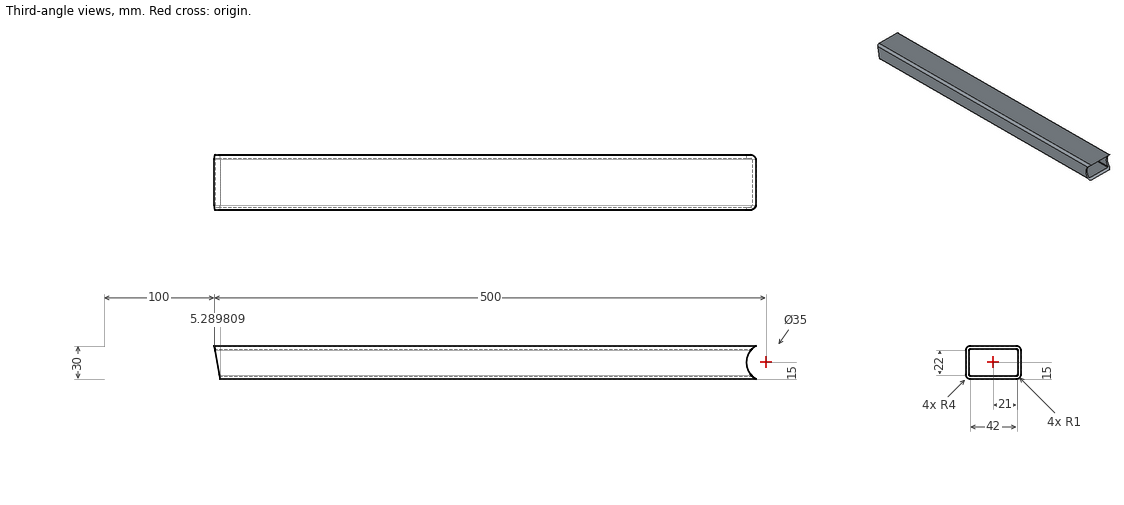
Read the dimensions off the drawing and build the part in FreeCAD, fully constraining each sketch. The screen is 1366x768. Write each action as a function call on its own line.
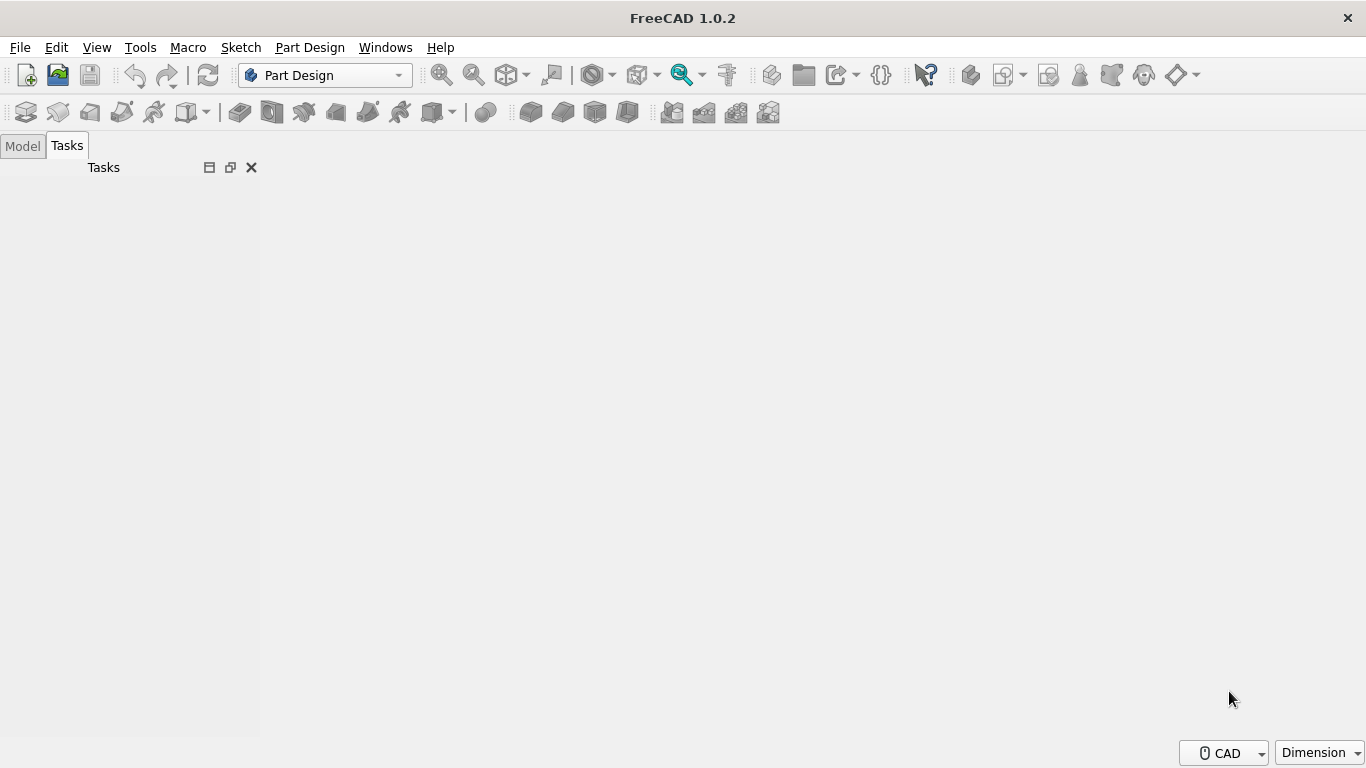
key(ctrl+n)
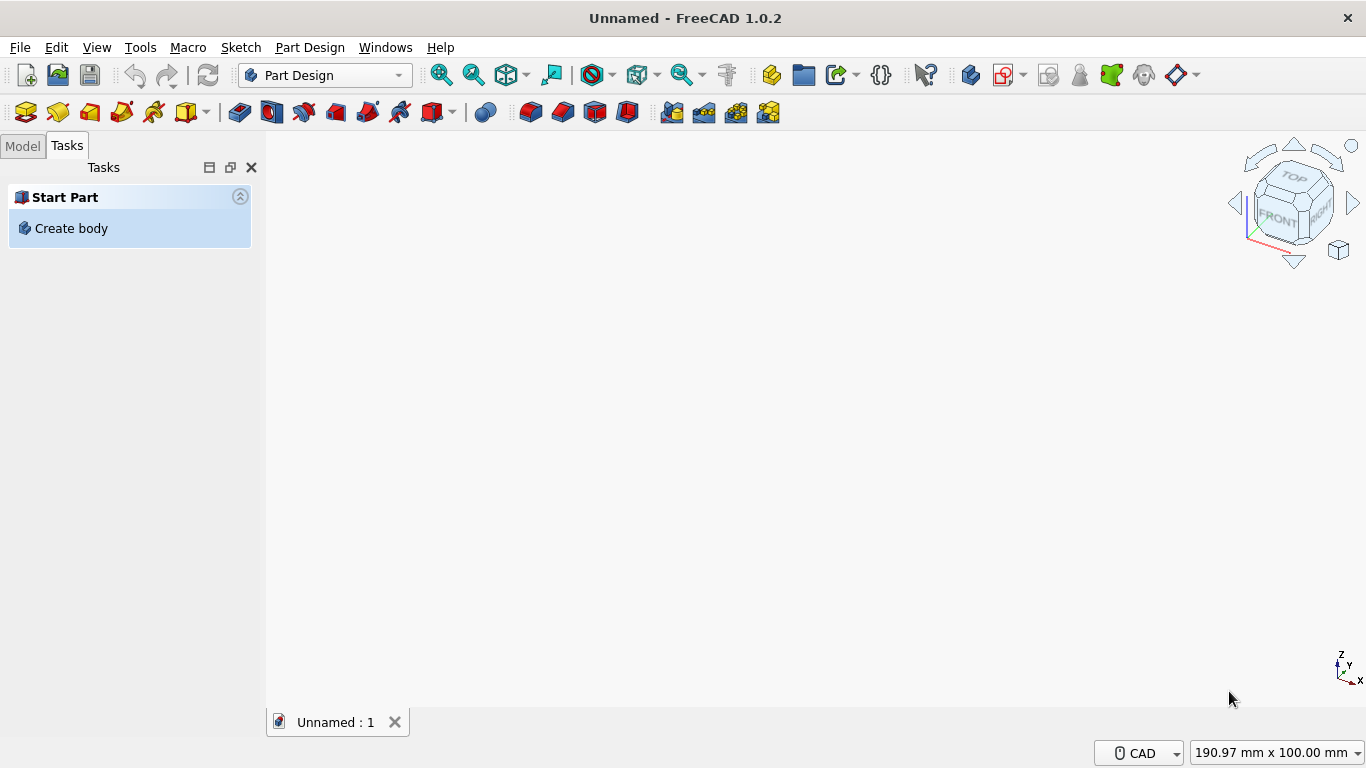
click(1004, 76)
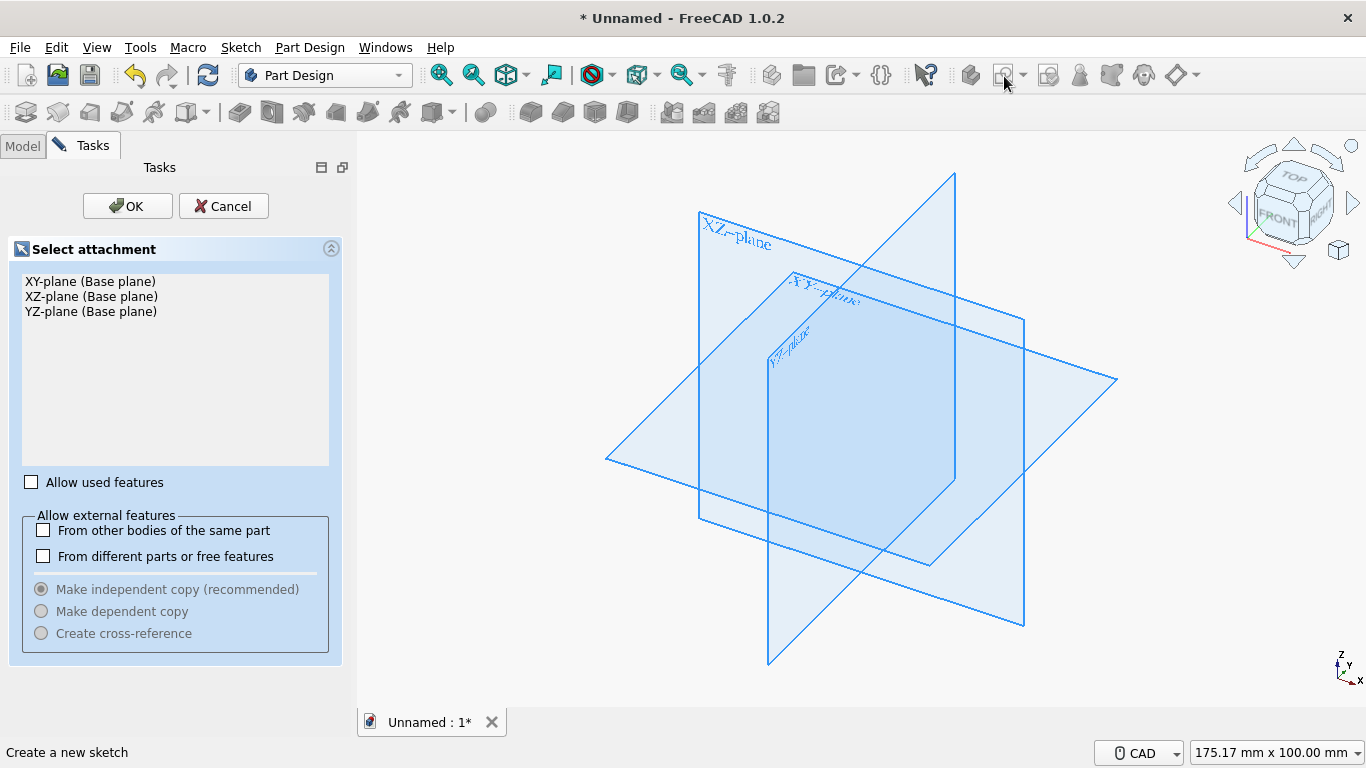
click(82, 312)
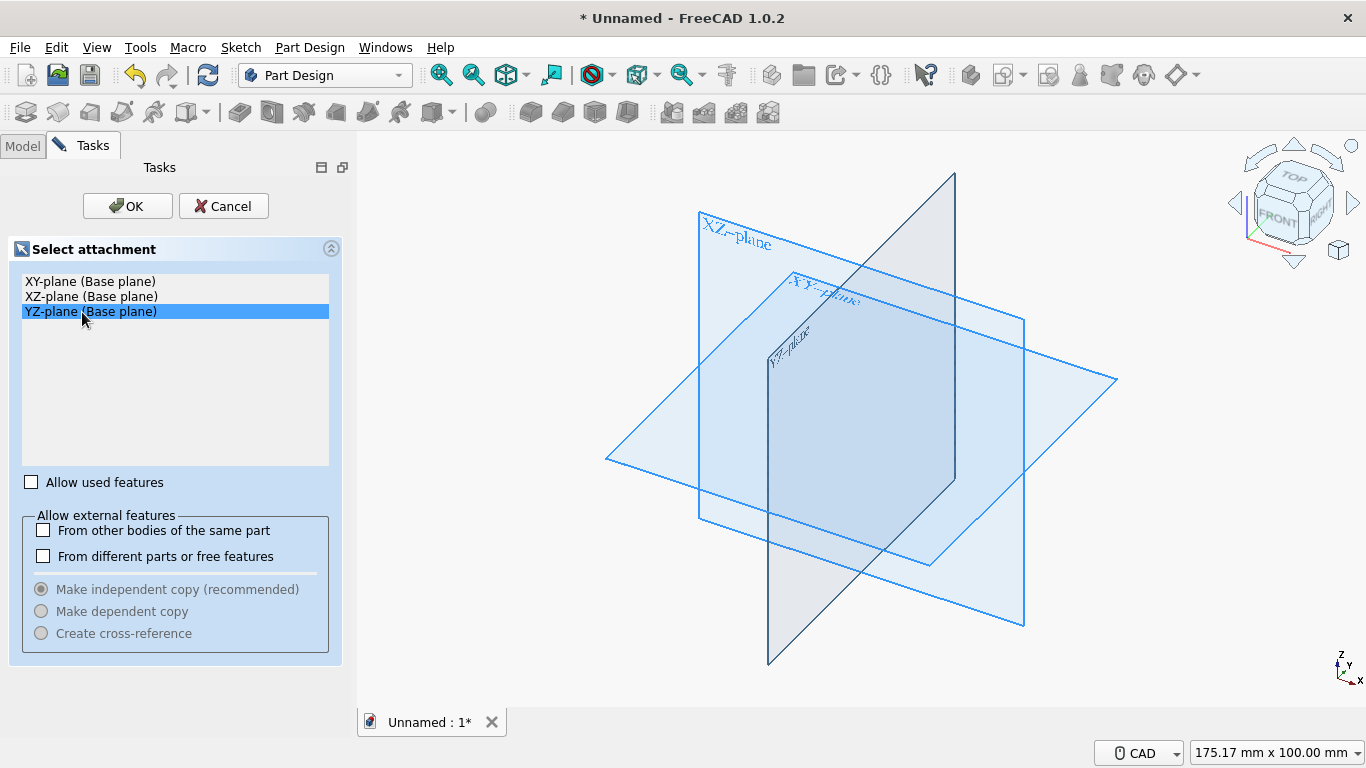
click(128, 206)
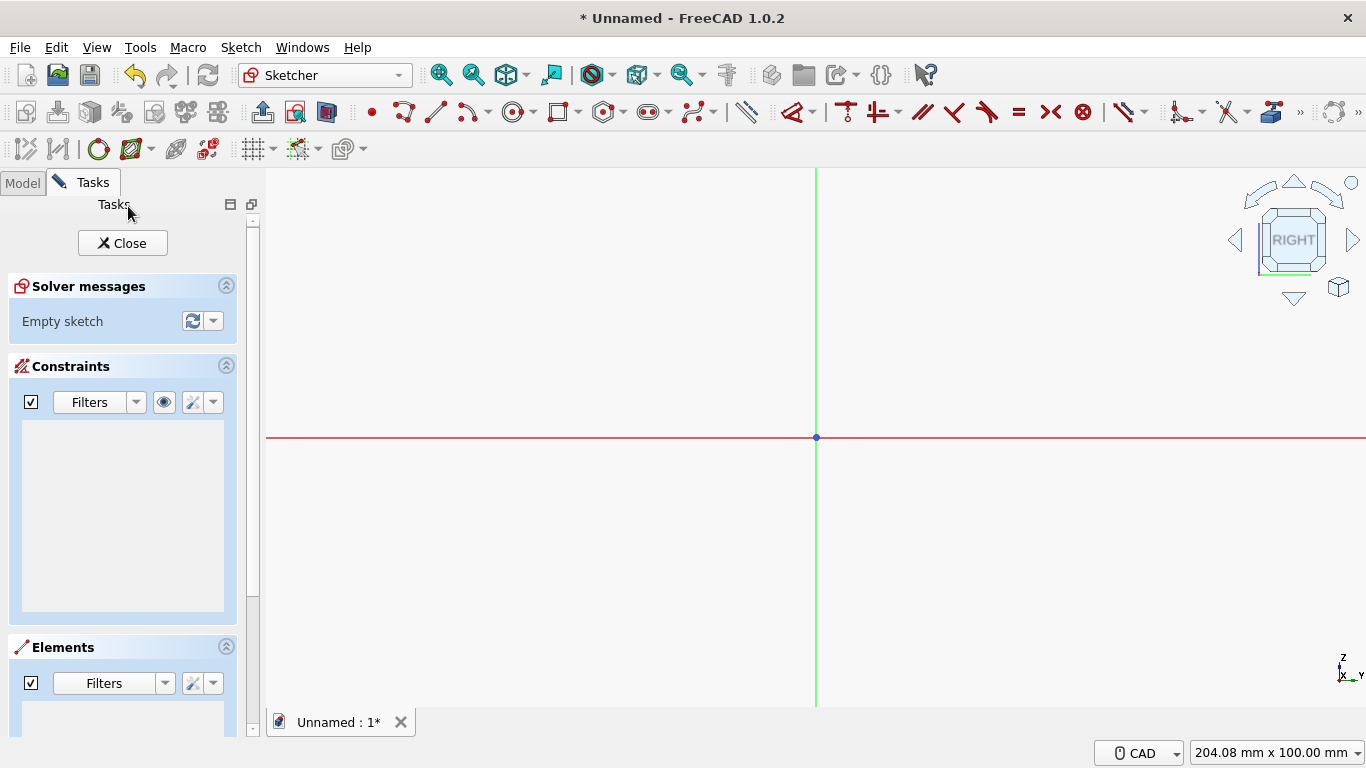
scroll(872, 438, up, 4)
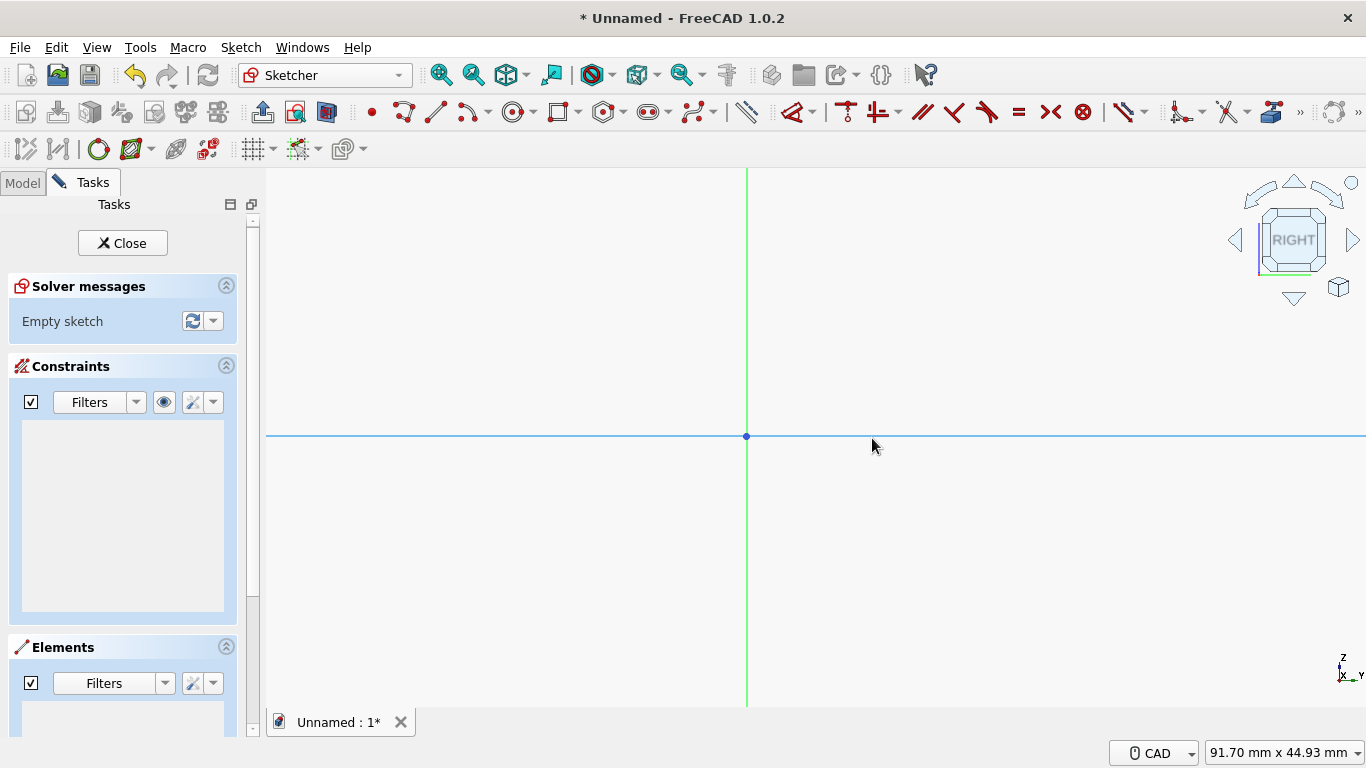
key(g)
key(l)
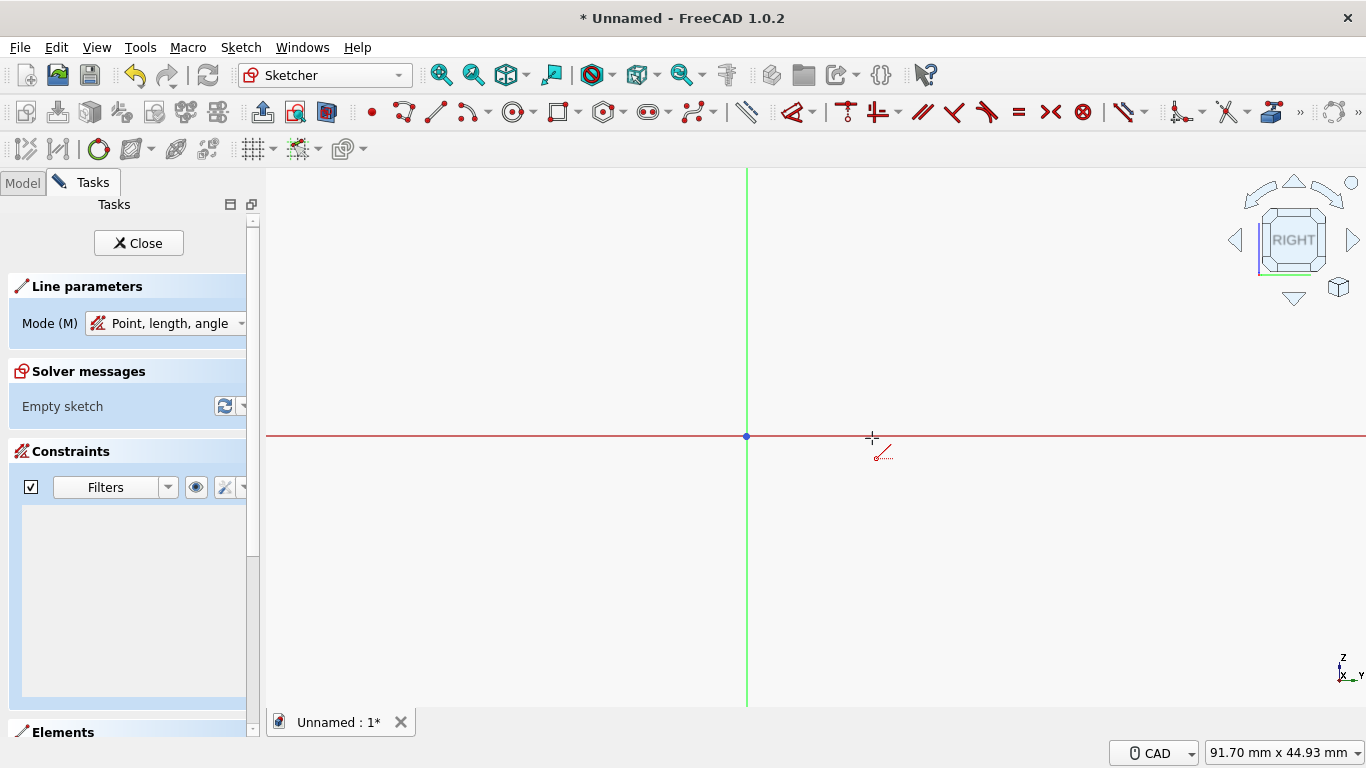
click(999, 616)
click(495, 616)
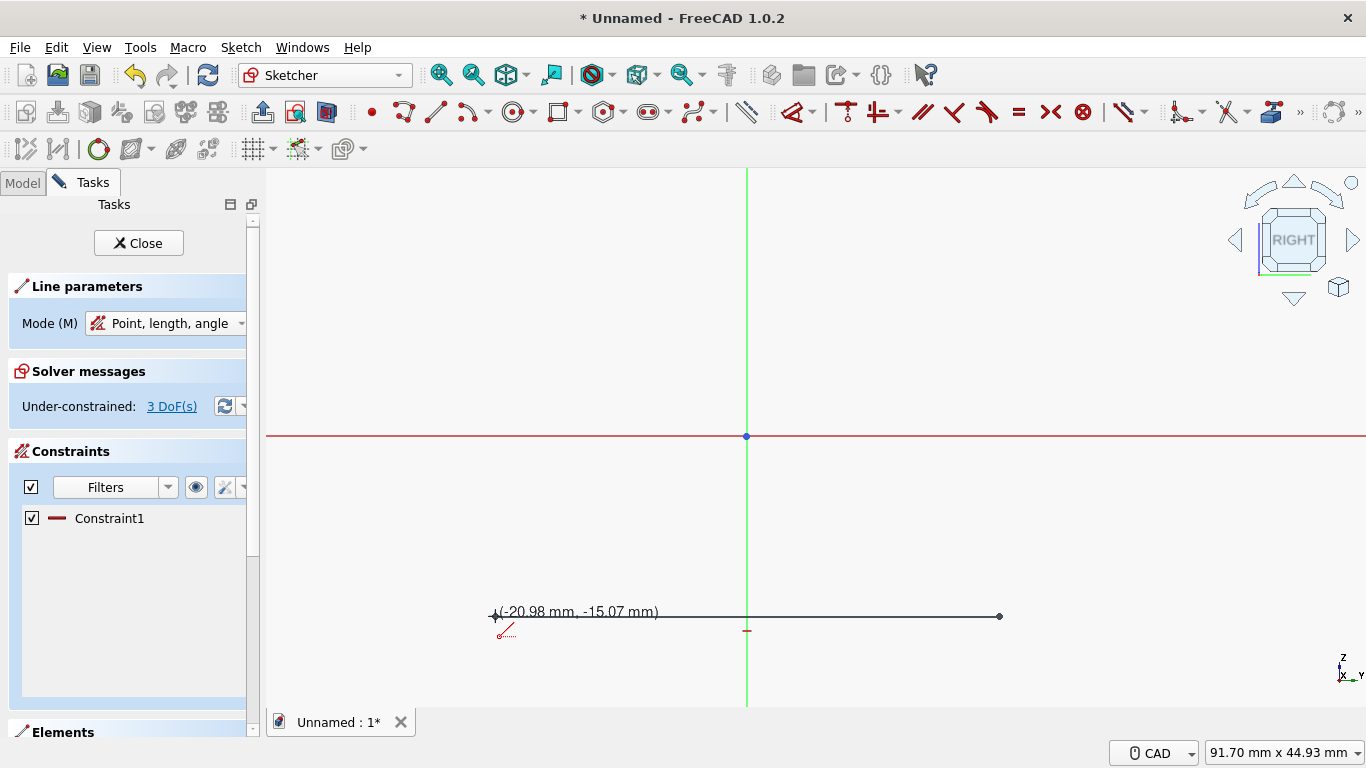
click(447, 568)
click(447, 304)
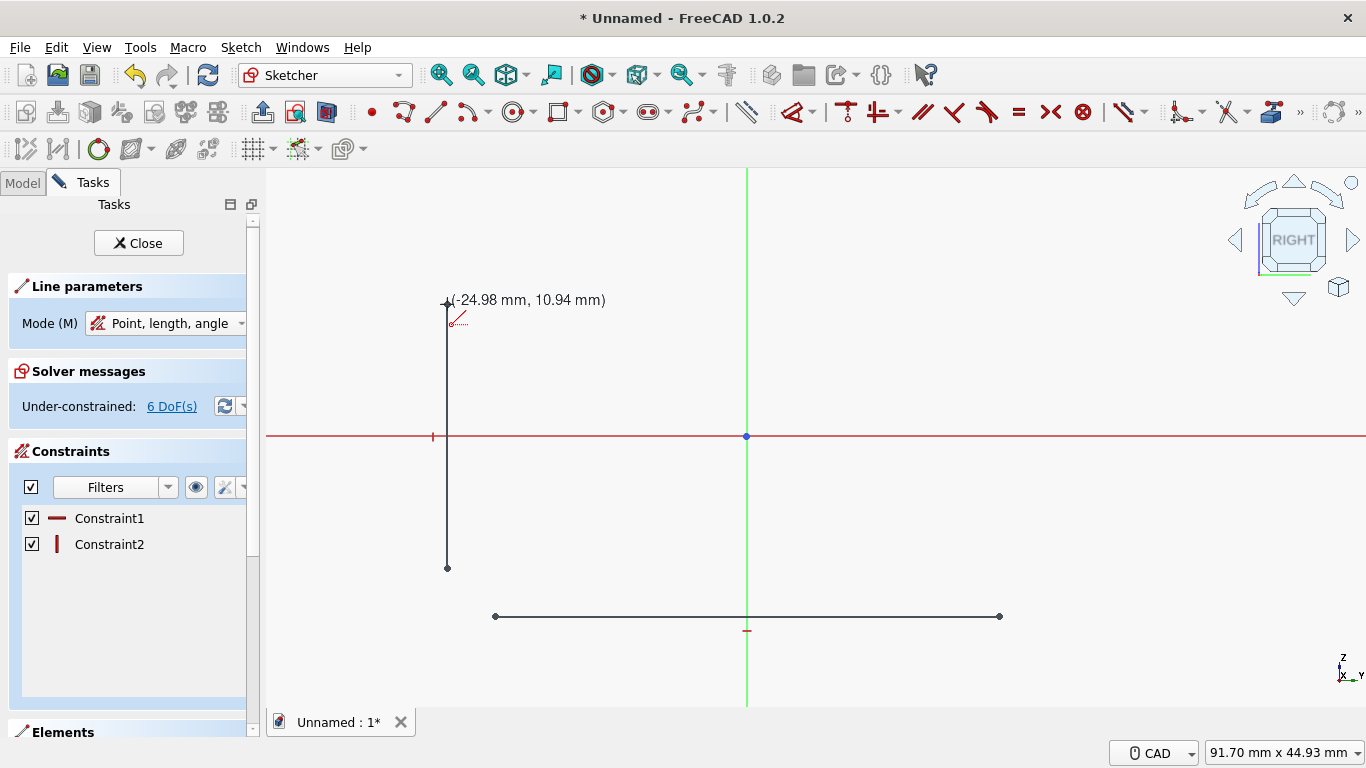
click(495, 256)
click(999, 256)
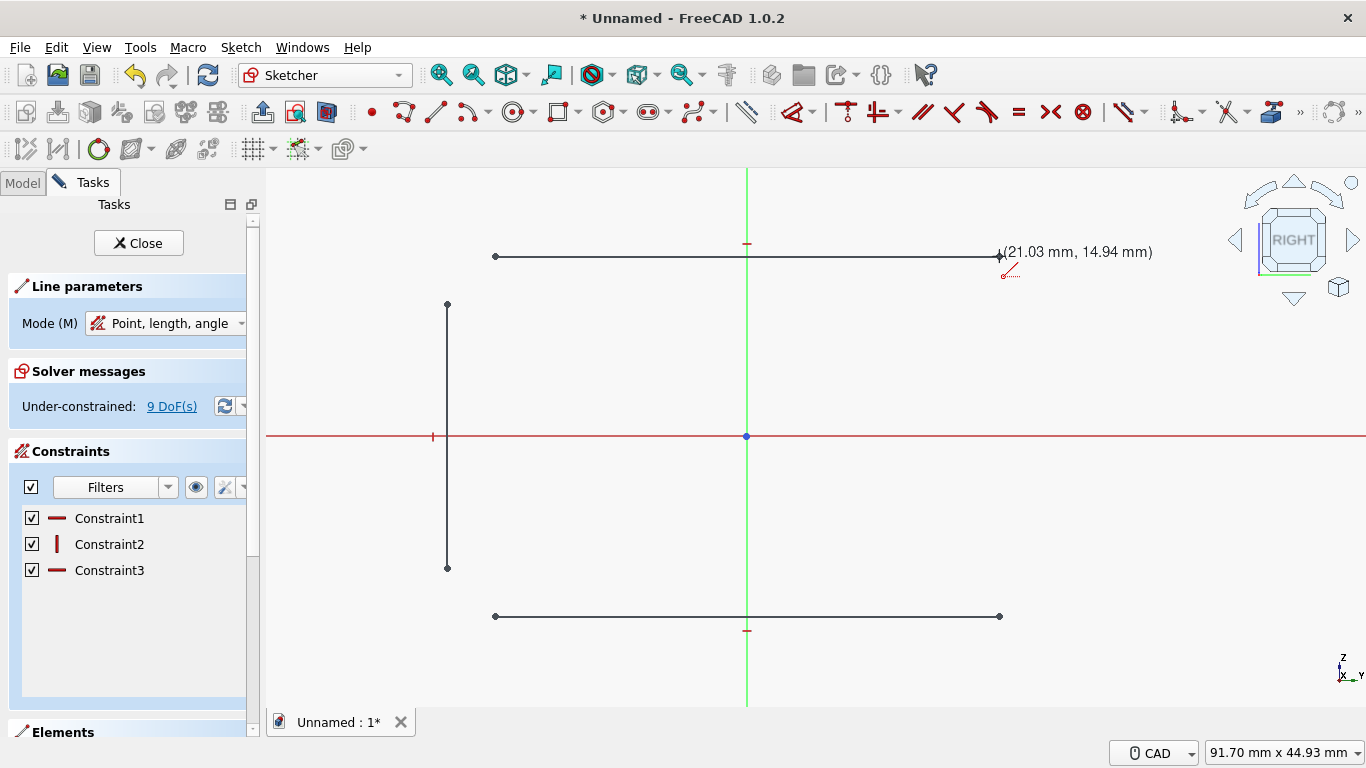
click(1047, 304)
click(1047, 568)